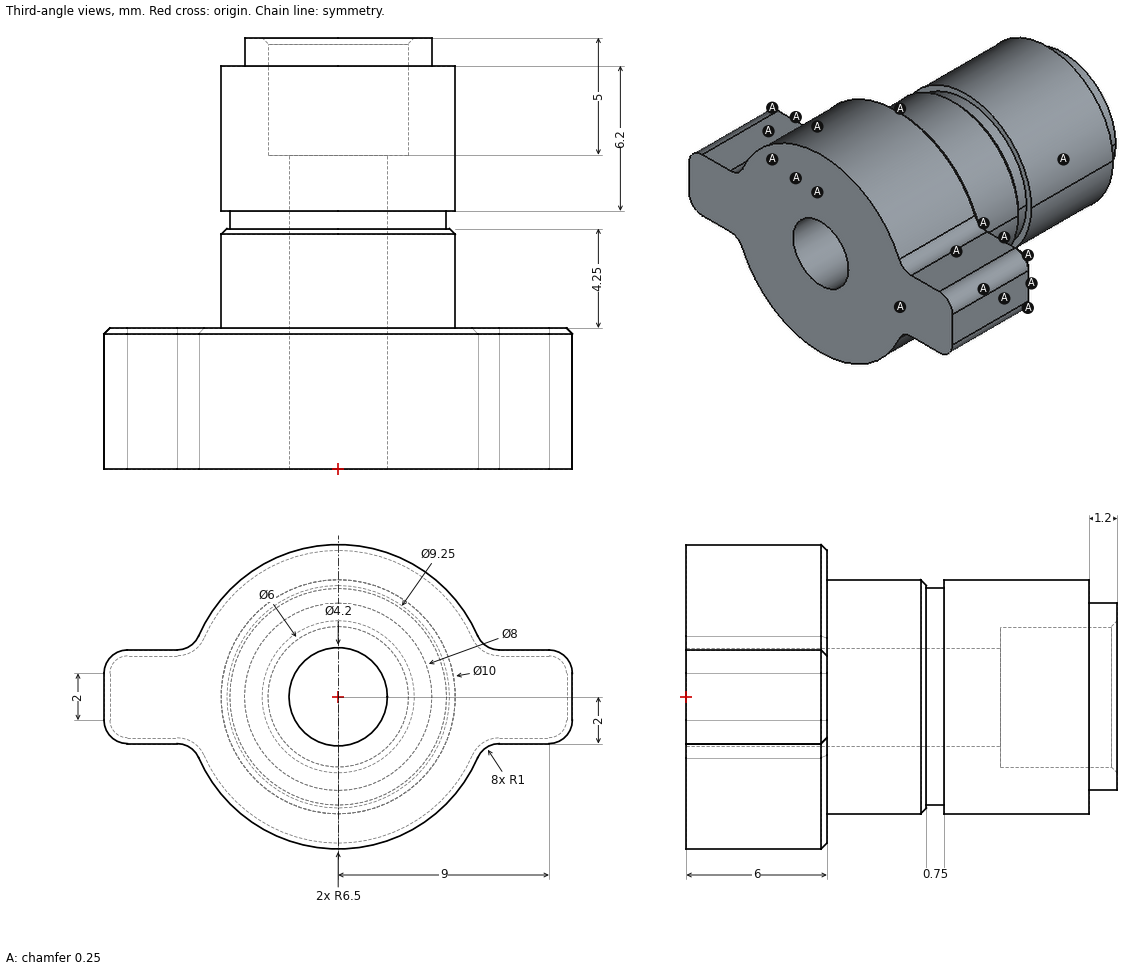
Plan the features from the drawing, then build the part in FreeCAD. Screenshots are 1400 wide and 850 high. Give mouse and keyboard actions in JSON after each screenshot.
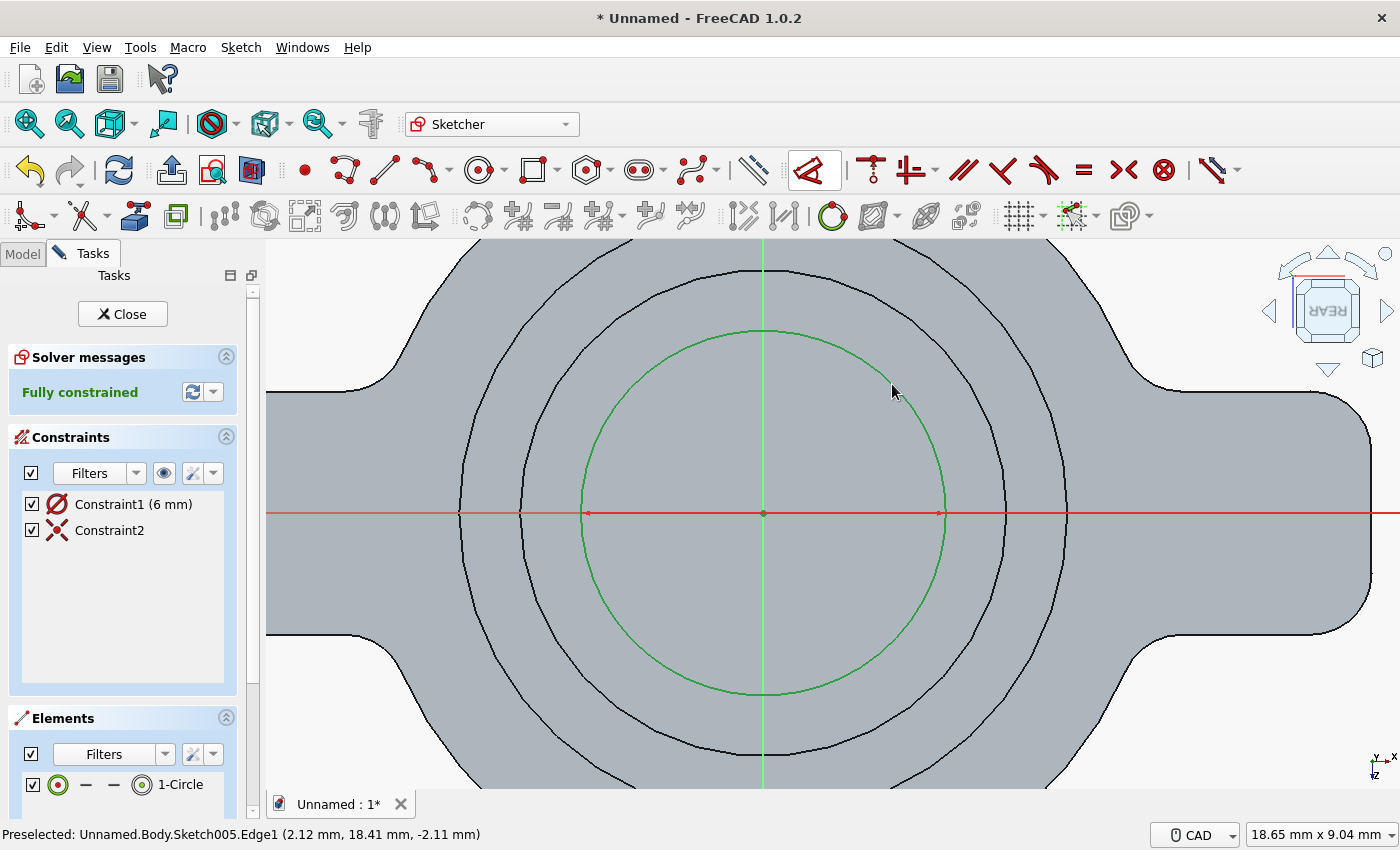
{"action": "left_click", "coordinate": [123, 314]}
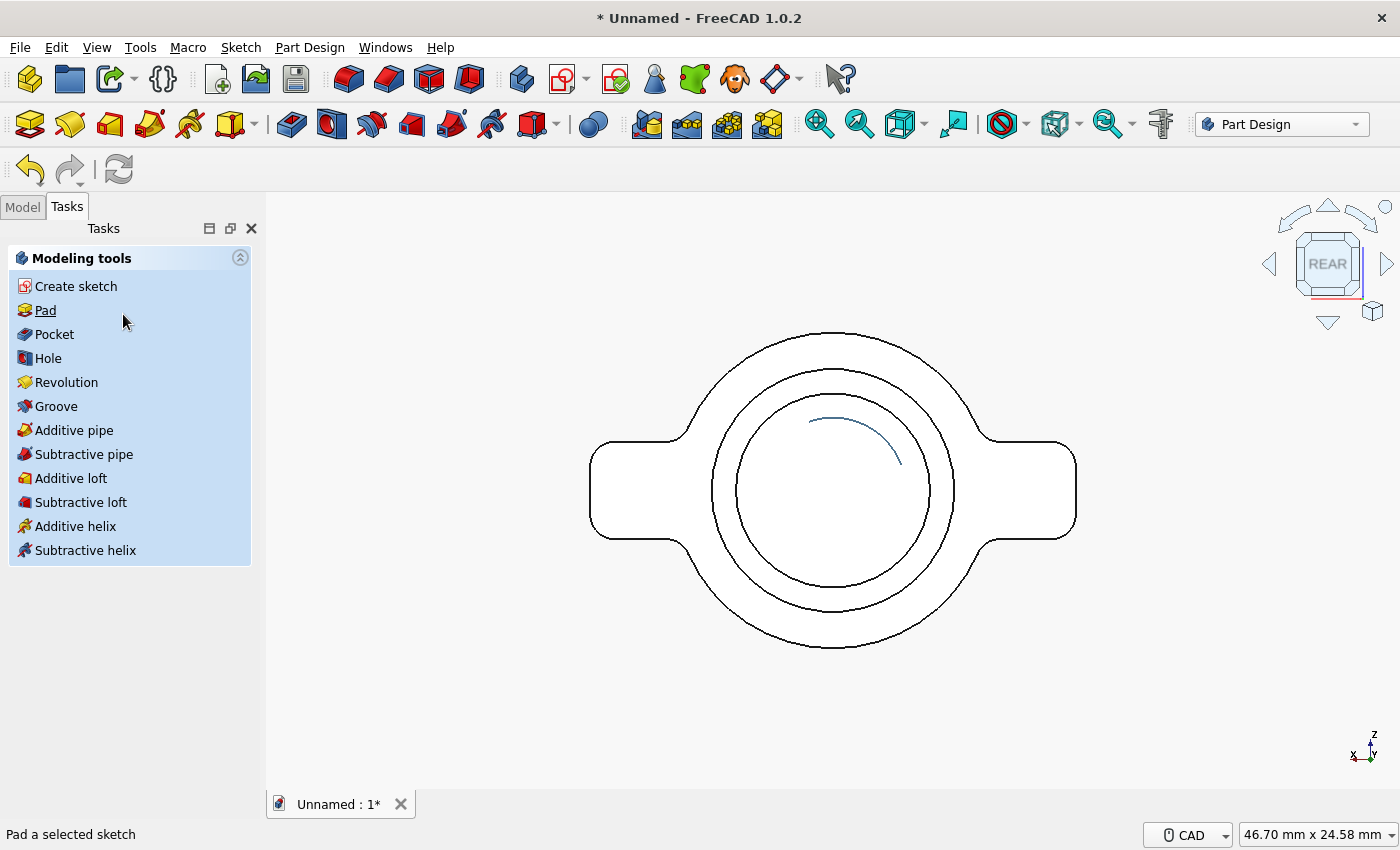
{"action": "left_click", "coordinate": [292, 124]}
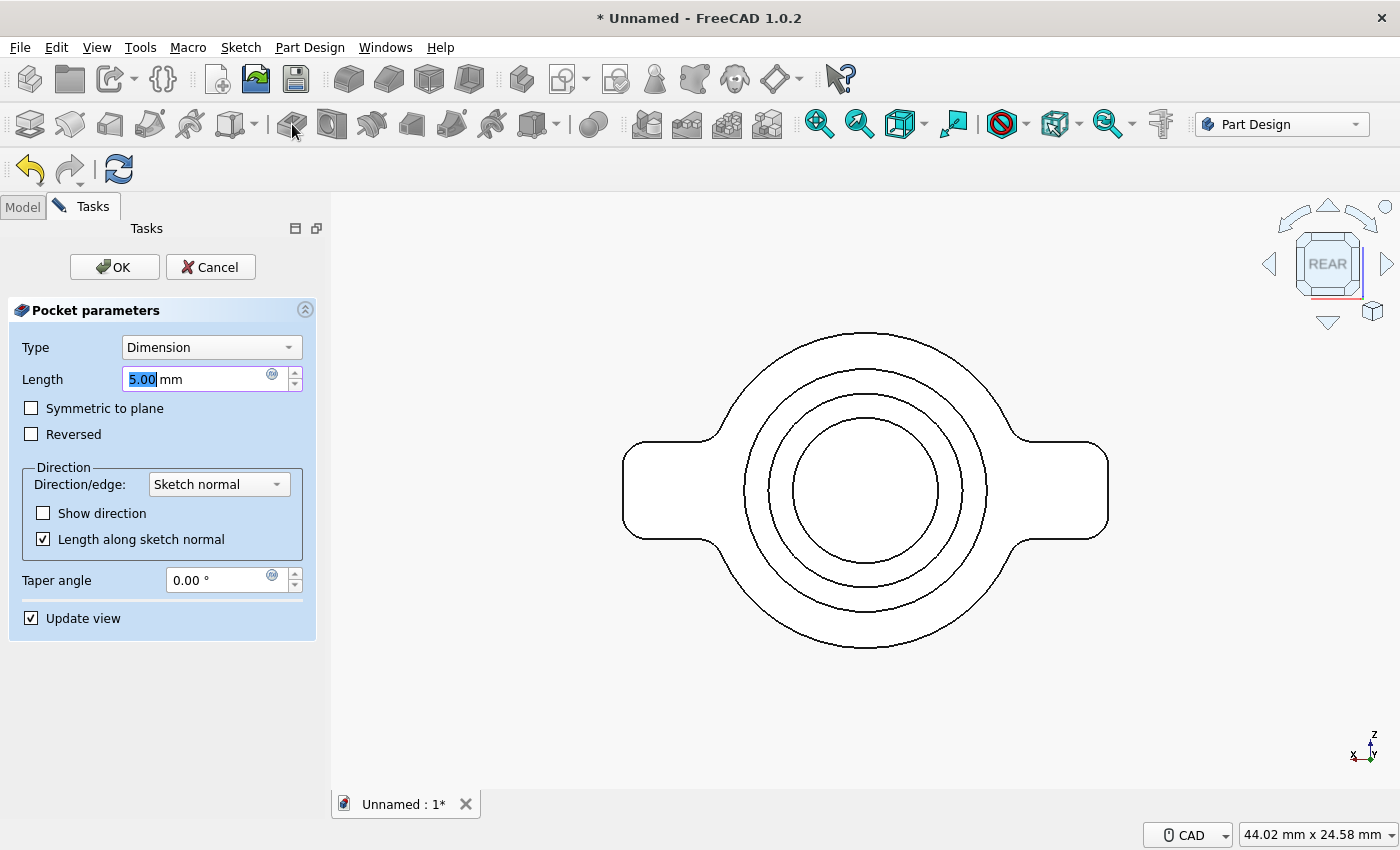
{"action": "type", "text": "5"}
{"action": "key", "text": "Tab"}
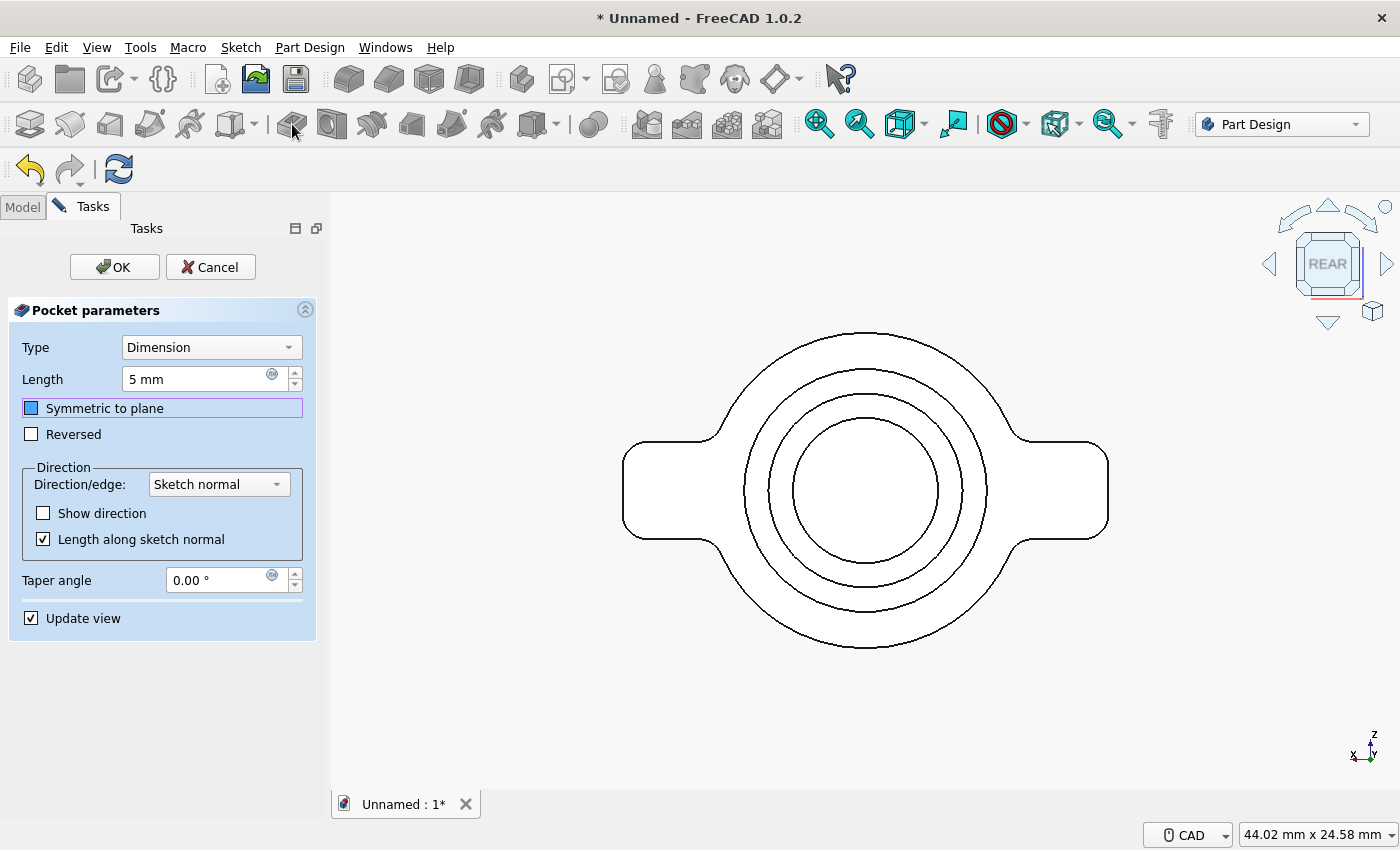
{"action": "left_click", "coordinate": [115, 267]}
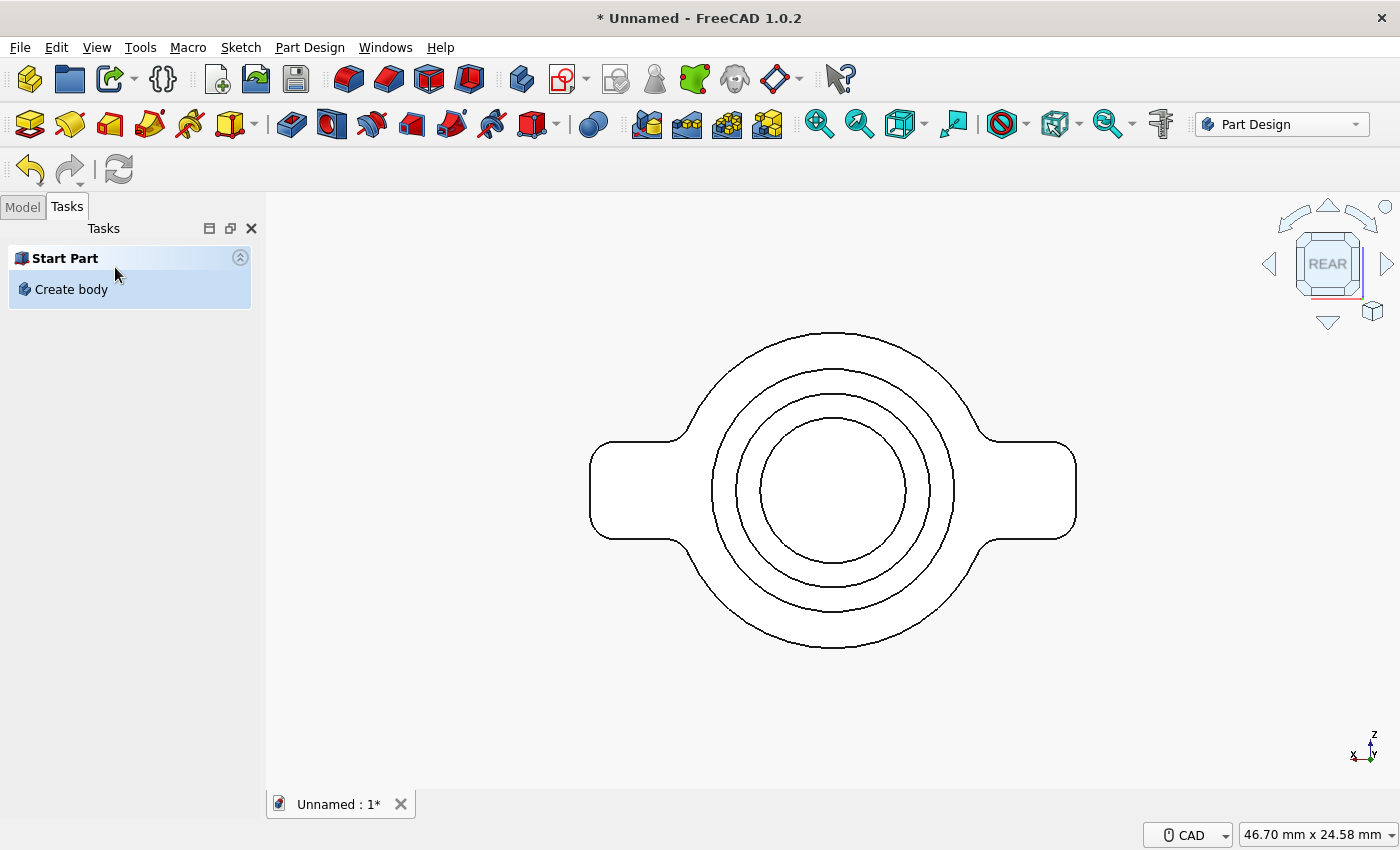
{"action": "left_click", "coordinate": [562, 80]}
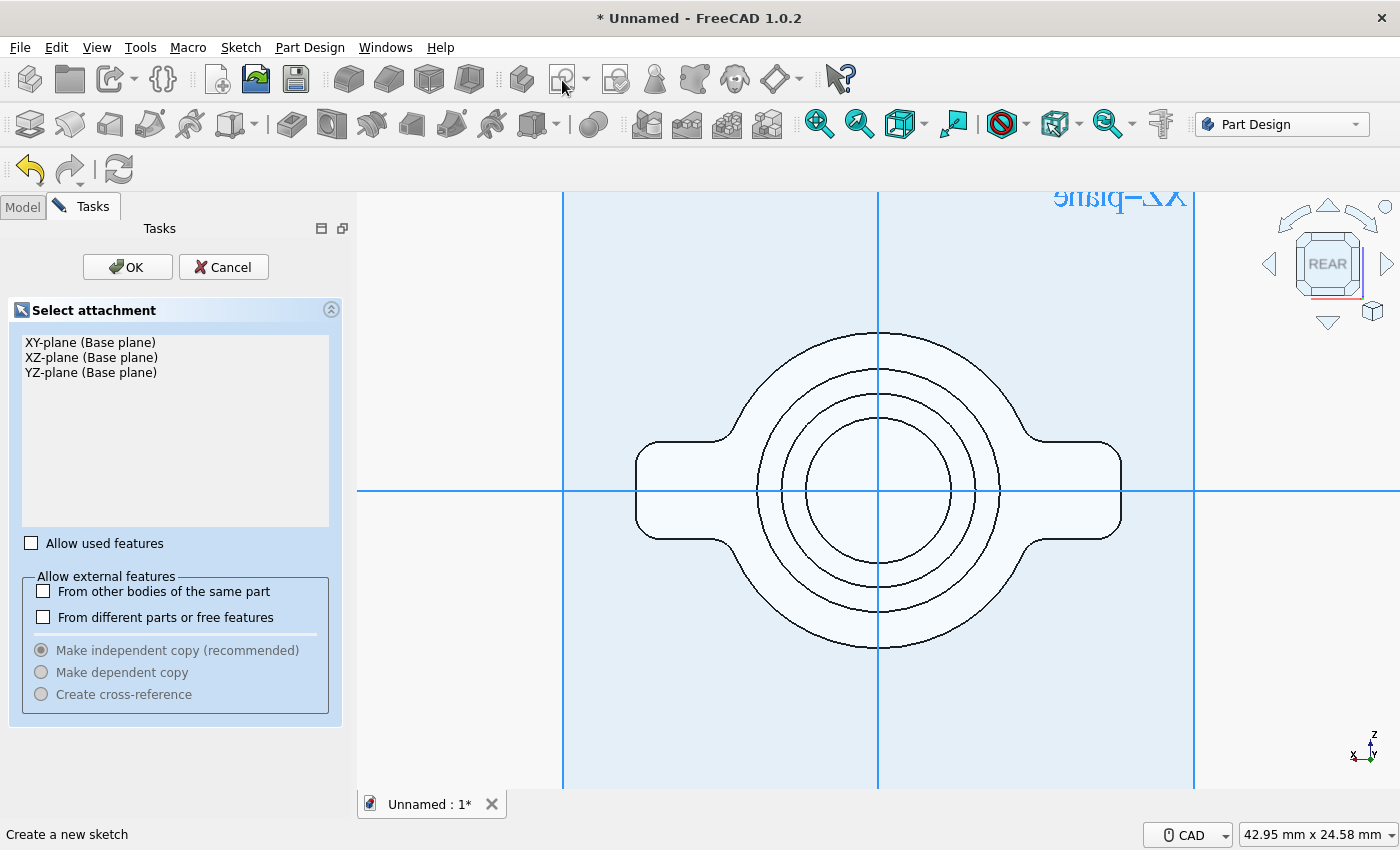
{"action": "left_click", "coordinate": [82, 358]}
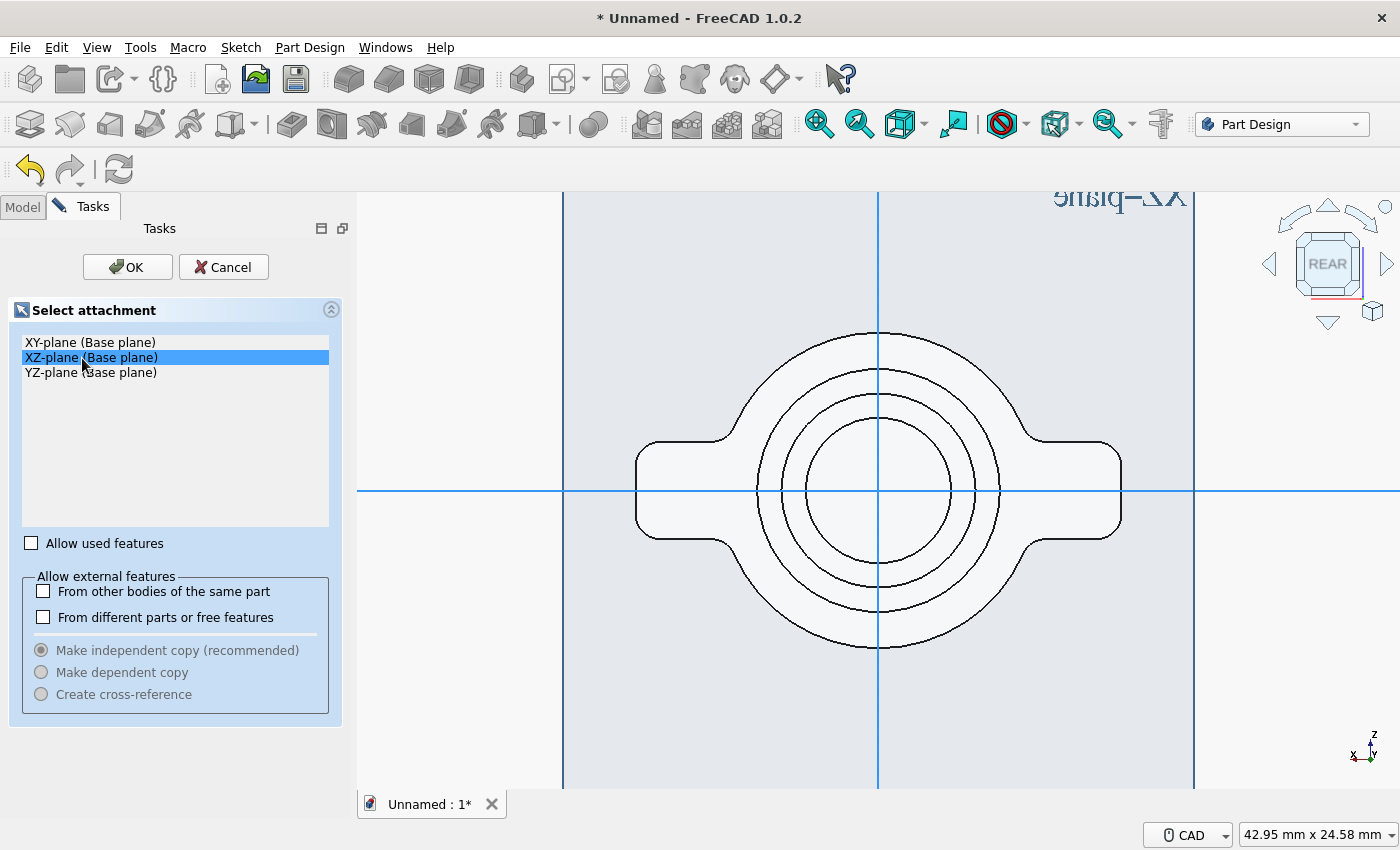
{"action": "left_click", "coordinate": [128, 267]}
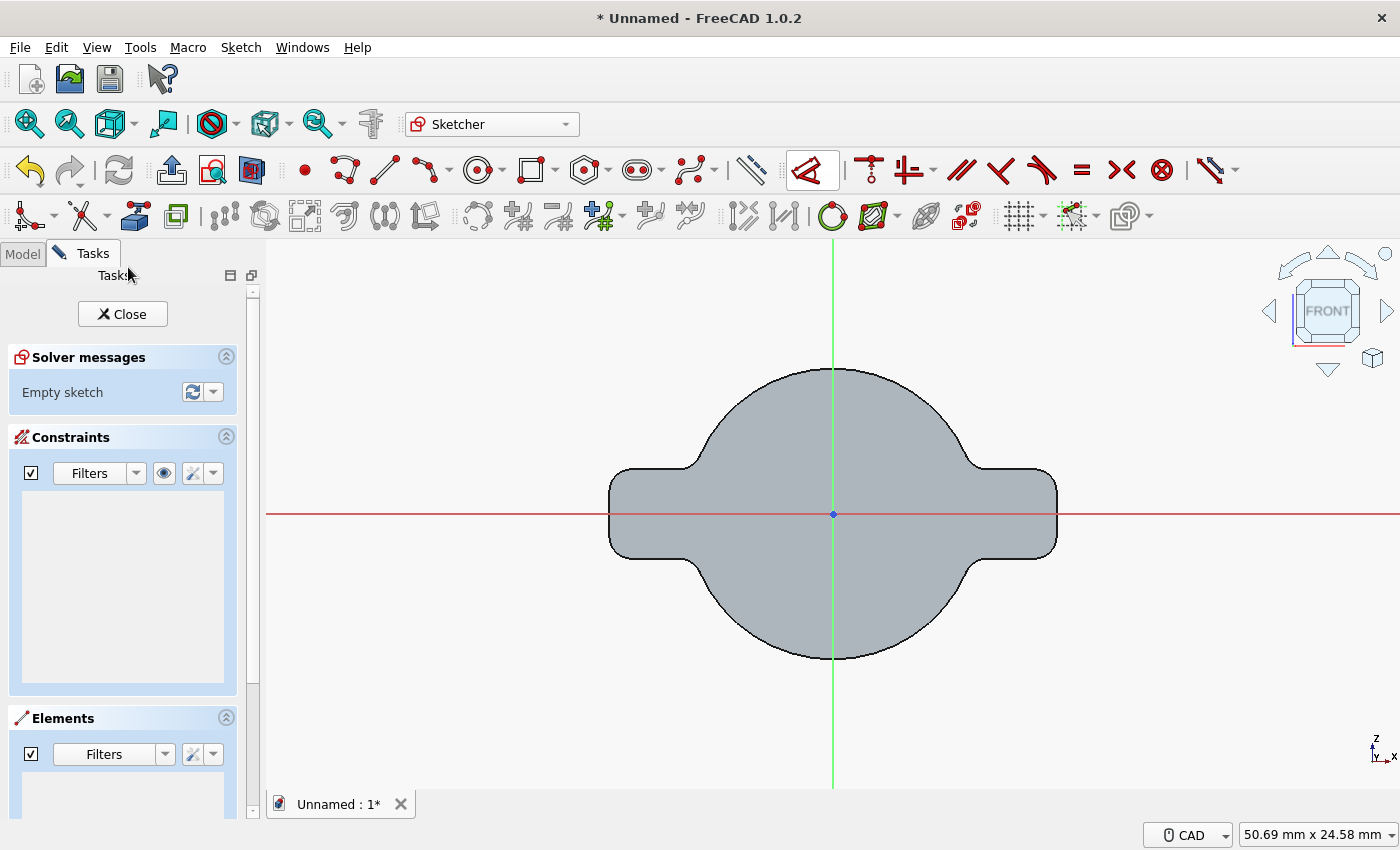
{"action": "scroll", "coordinate": [855, 514], "scroll_direction": "up", "scroll_amount": 7}